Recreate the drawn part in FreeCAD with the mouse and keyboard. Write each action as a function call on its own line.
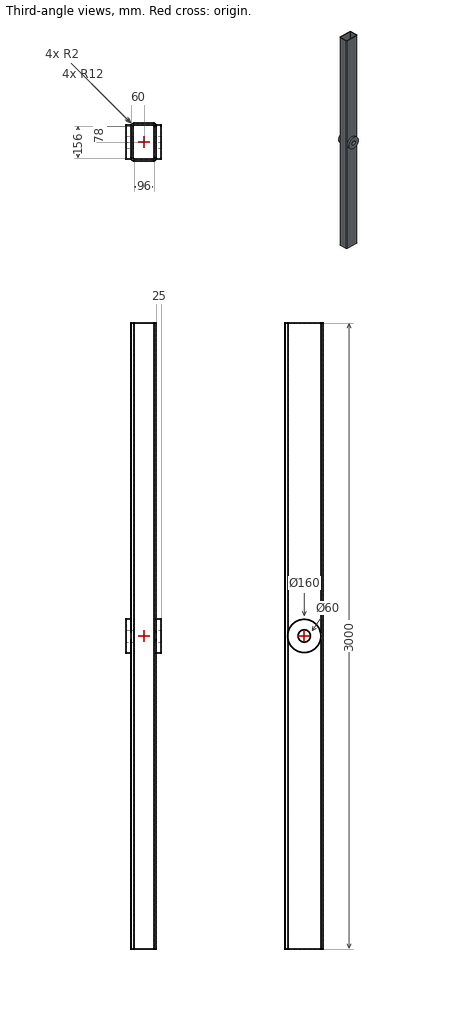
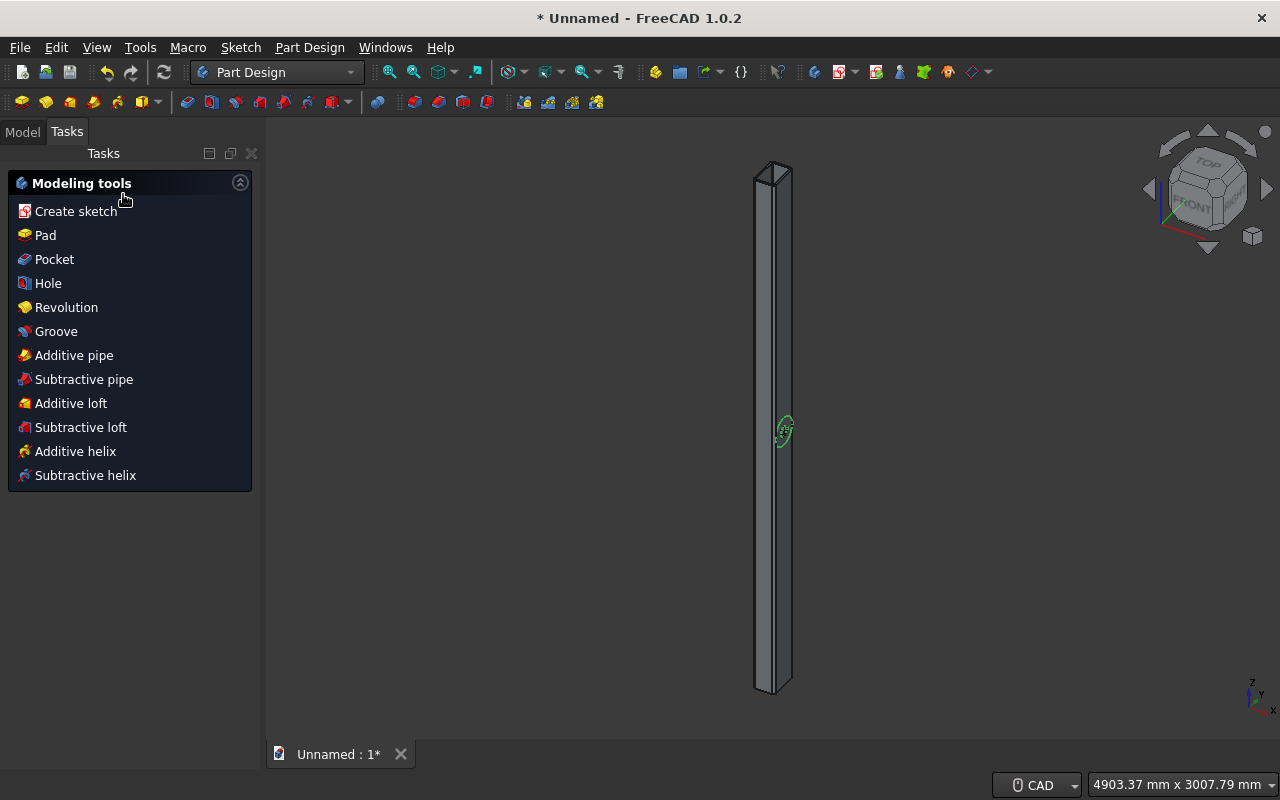
click(22, 102)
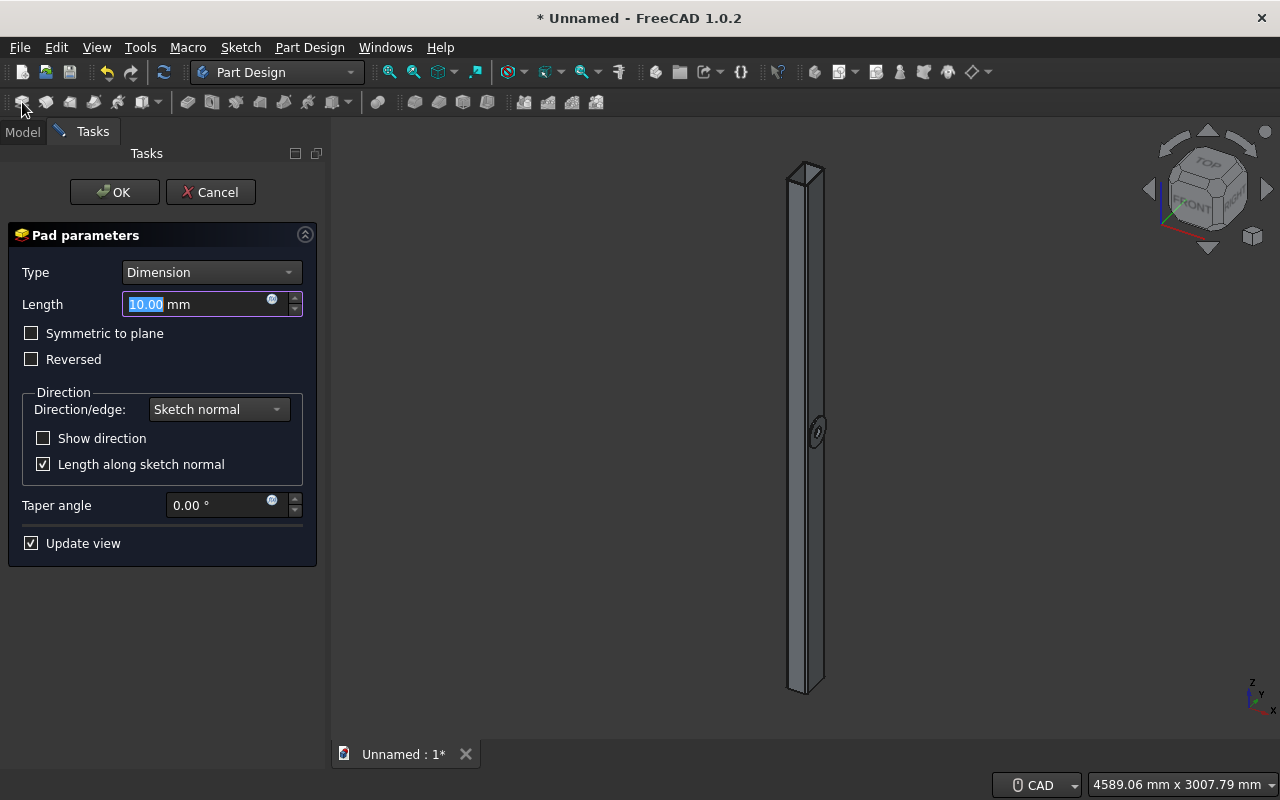
text(25)
key(Tab)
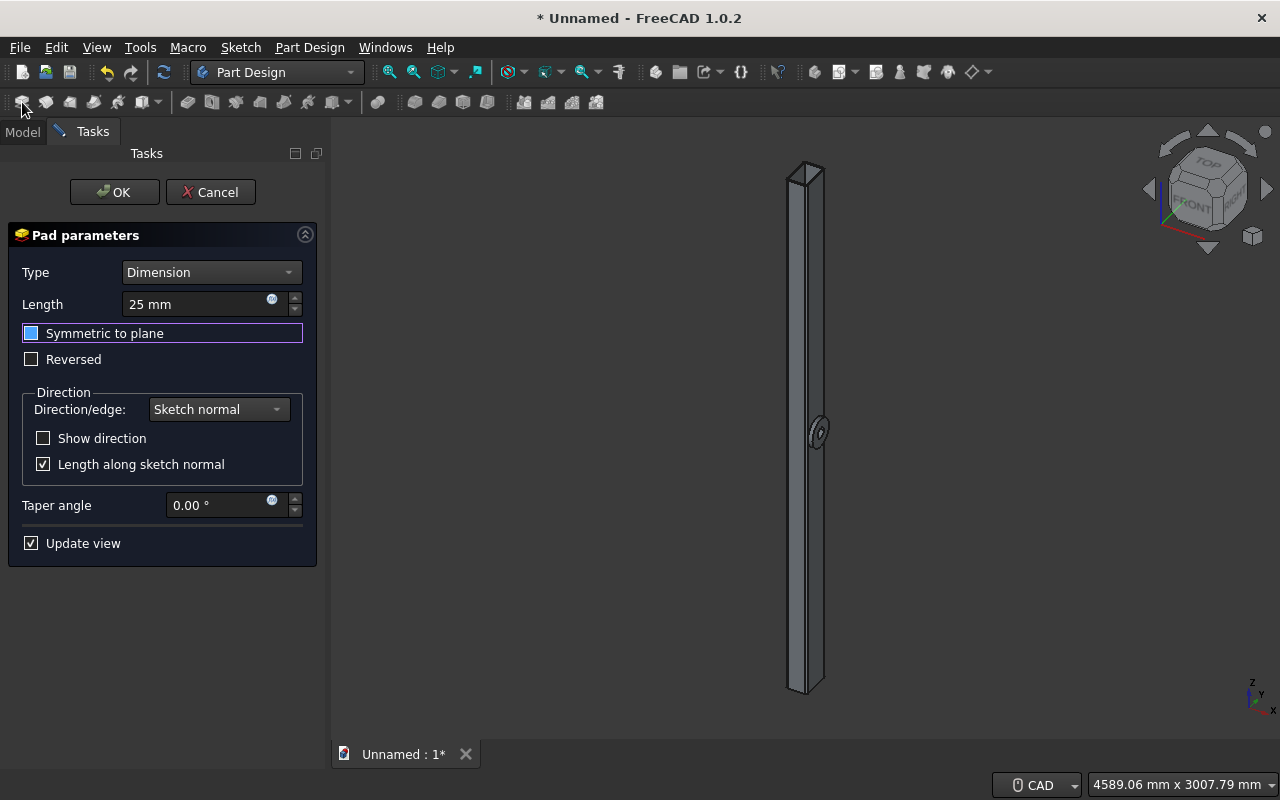
click(115, 192)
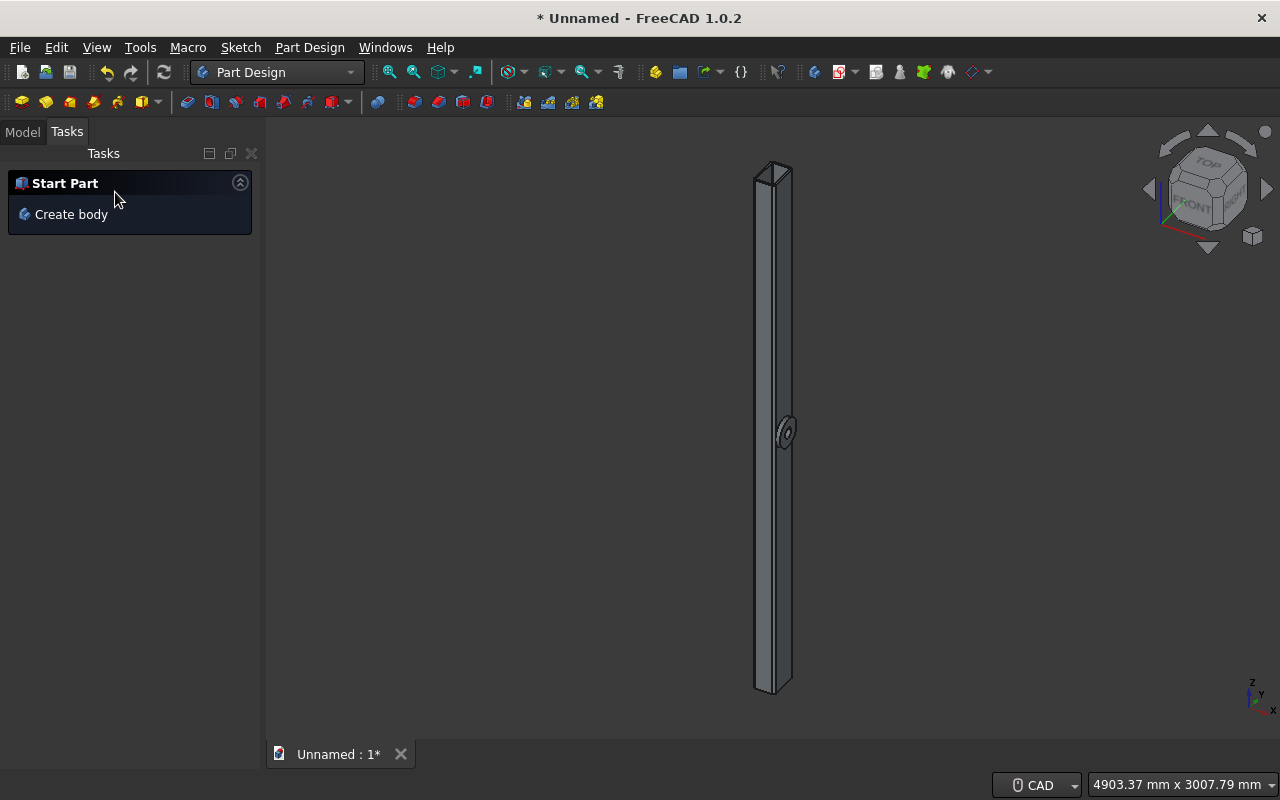
click(23, 131)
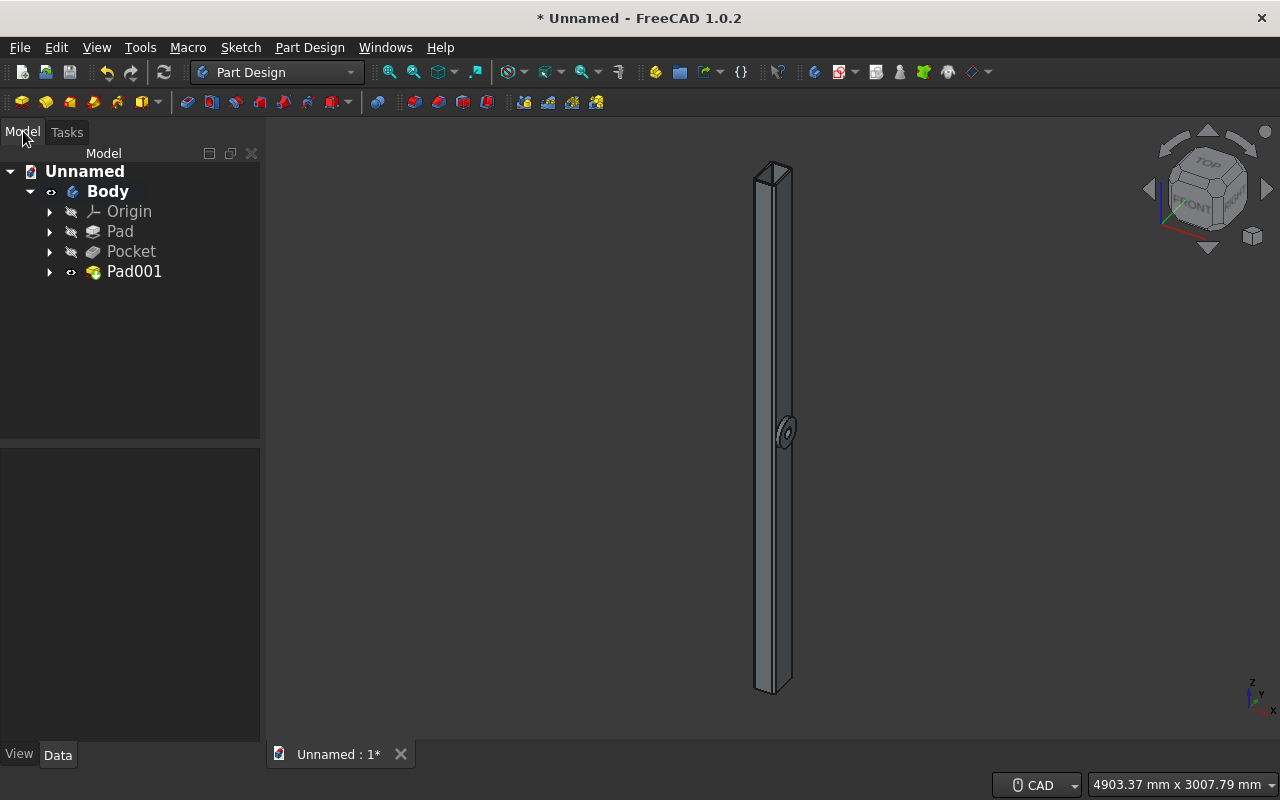
click(116, 272)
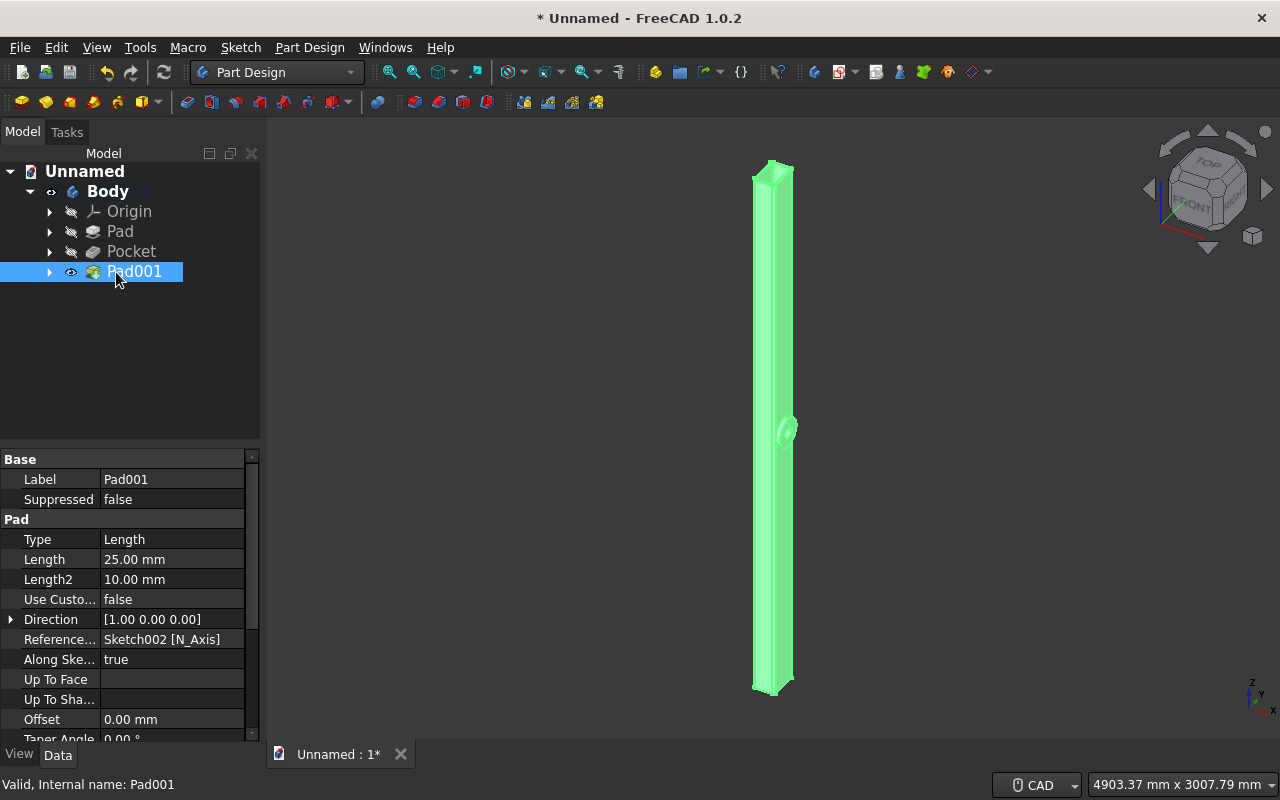
click(524, 102)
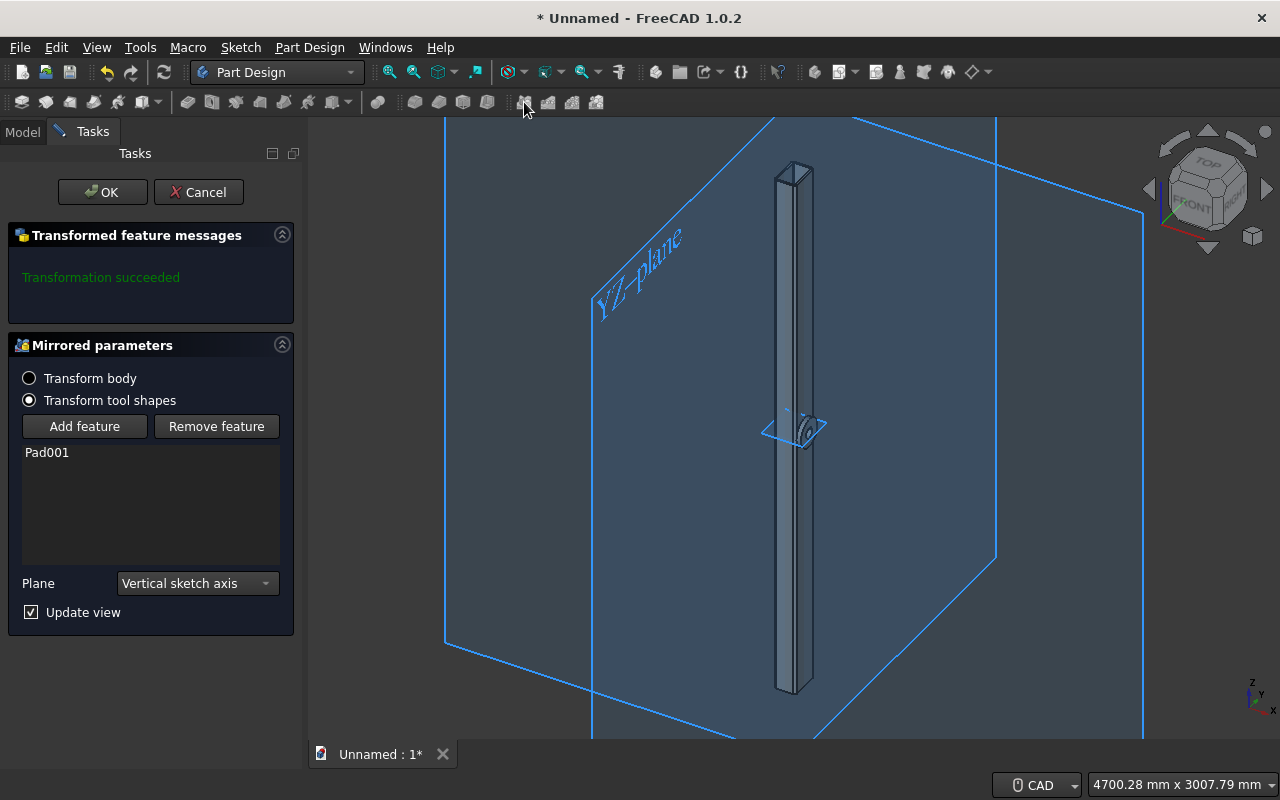
click(198, 584)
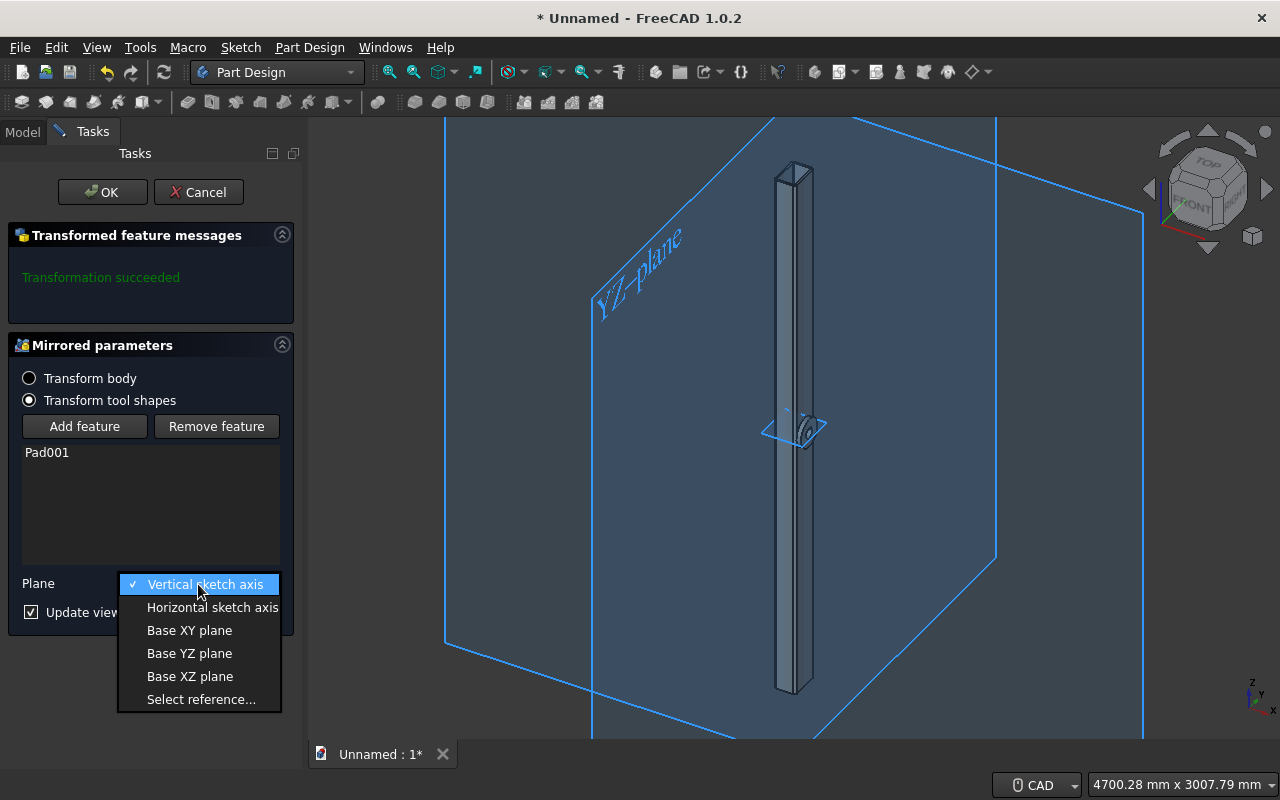
click(198, 654)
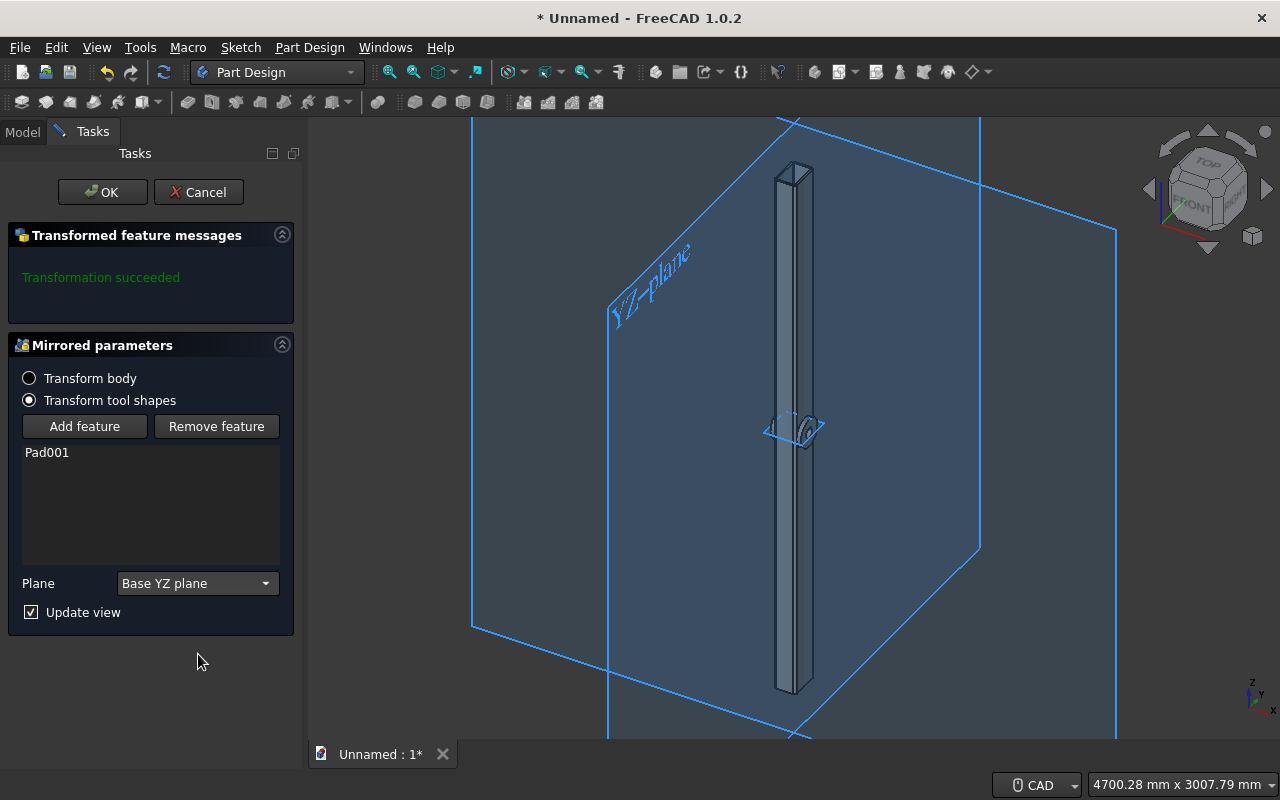
click(103, 192)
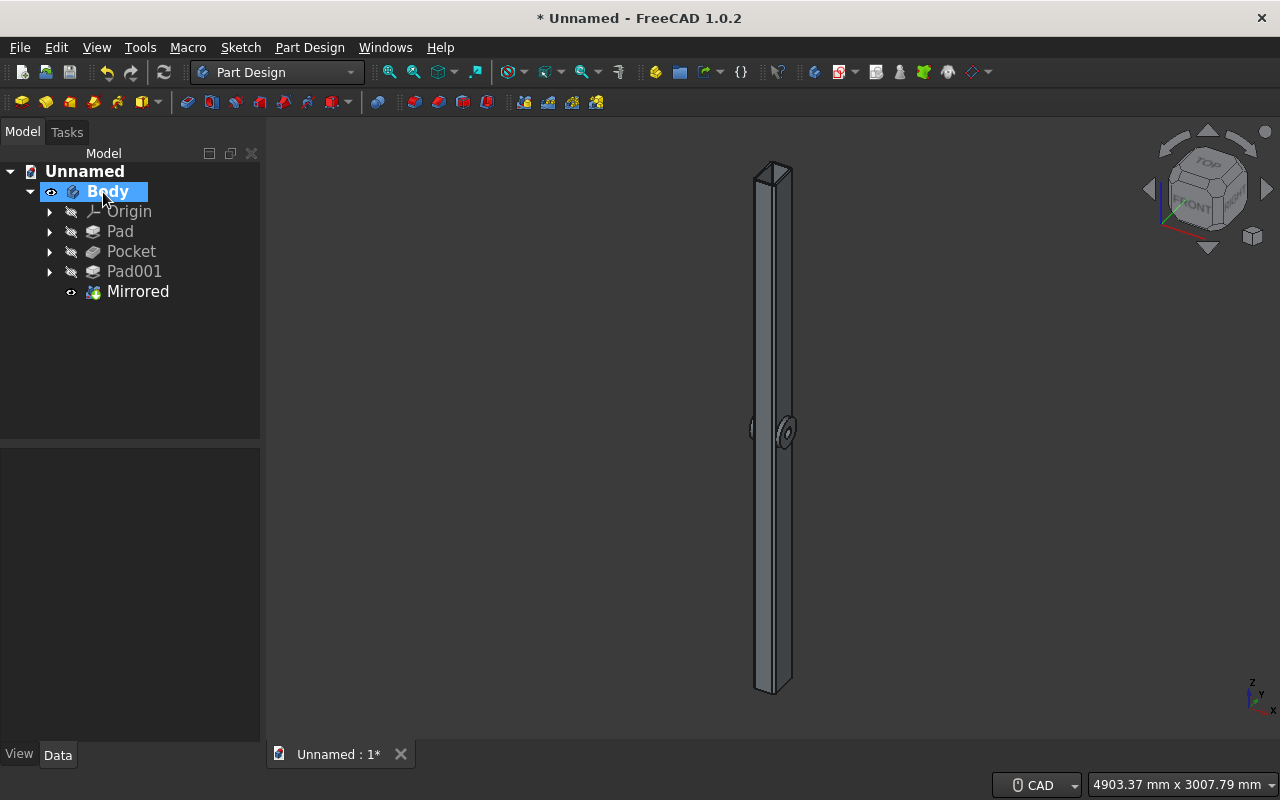
key(0)